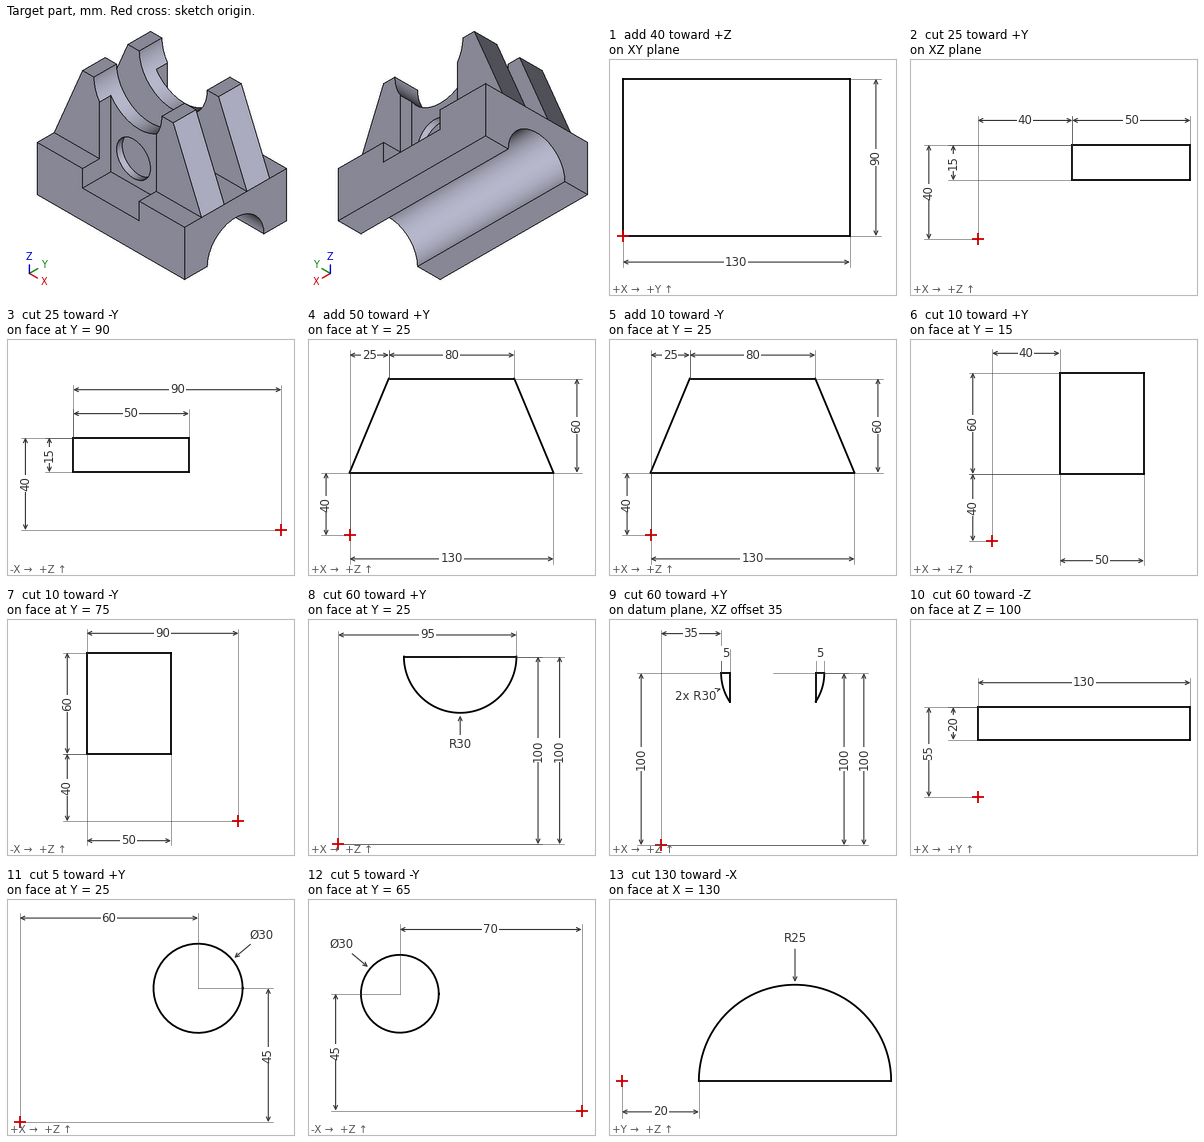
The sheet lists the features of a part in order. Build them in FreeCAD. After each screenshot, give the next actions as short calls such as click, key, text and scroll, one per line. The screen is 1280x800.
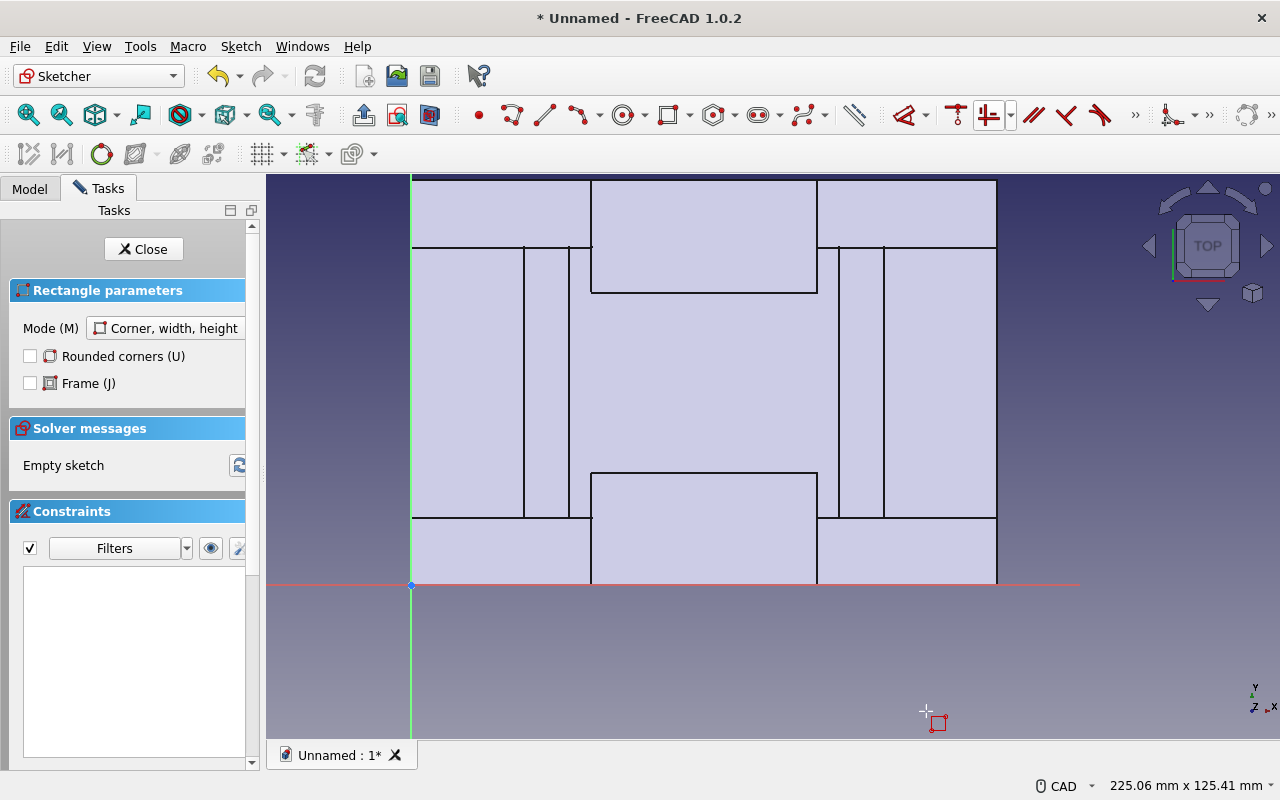
click(411, 338)
click(997, 428)
key(Escape)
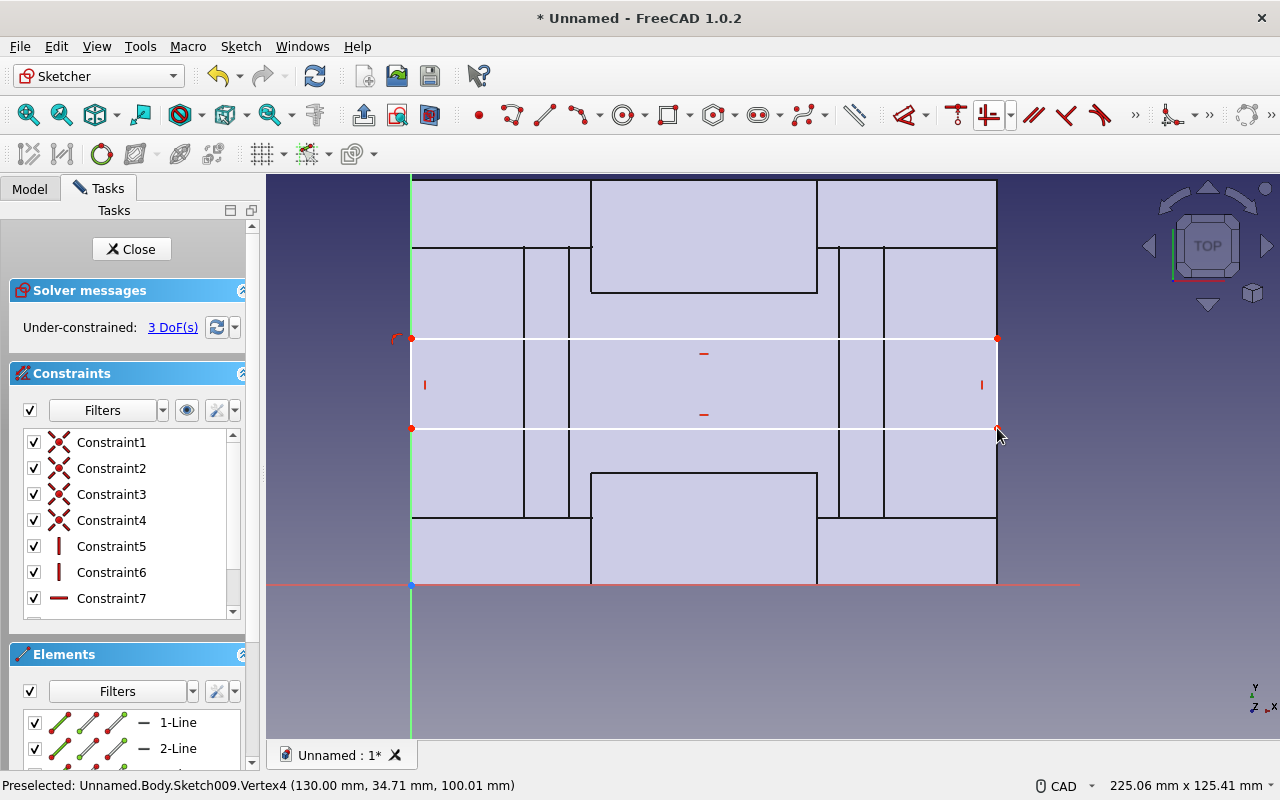
key(d)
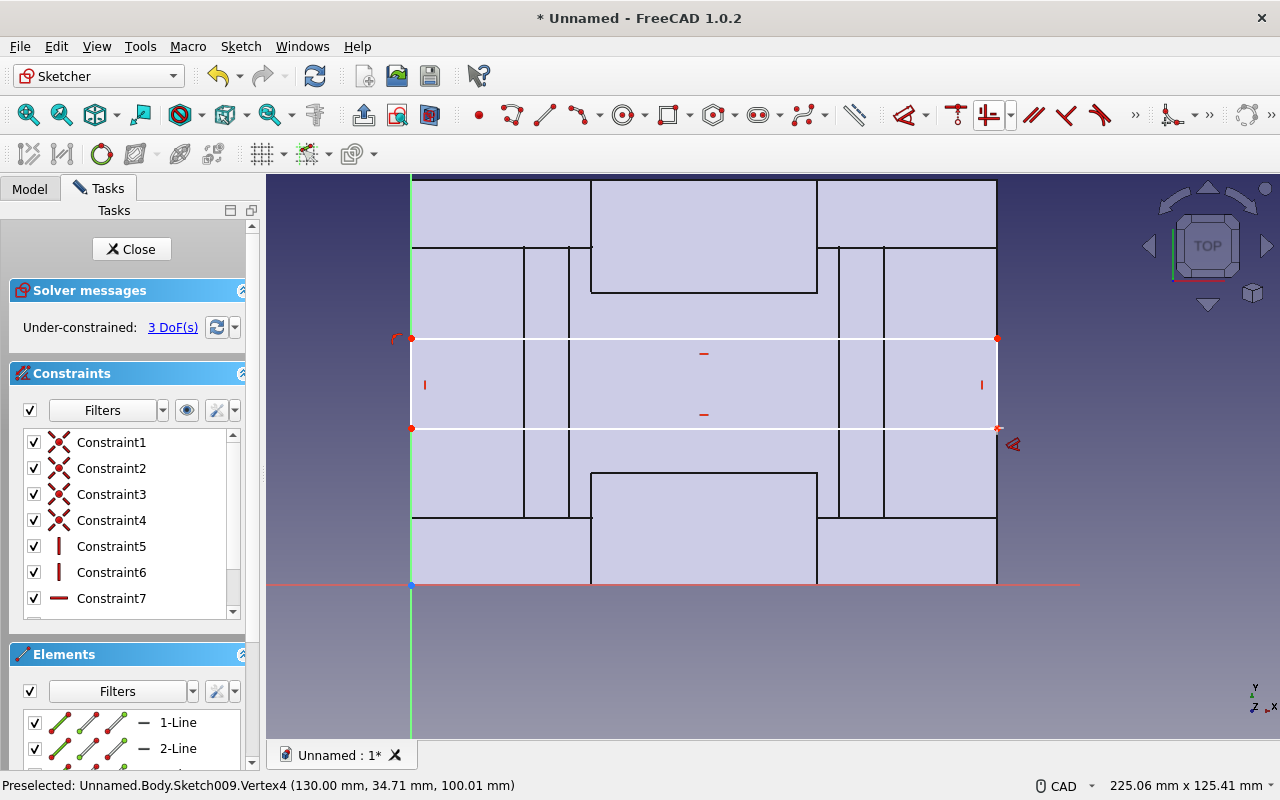
click(411, 366)
click(377, 384)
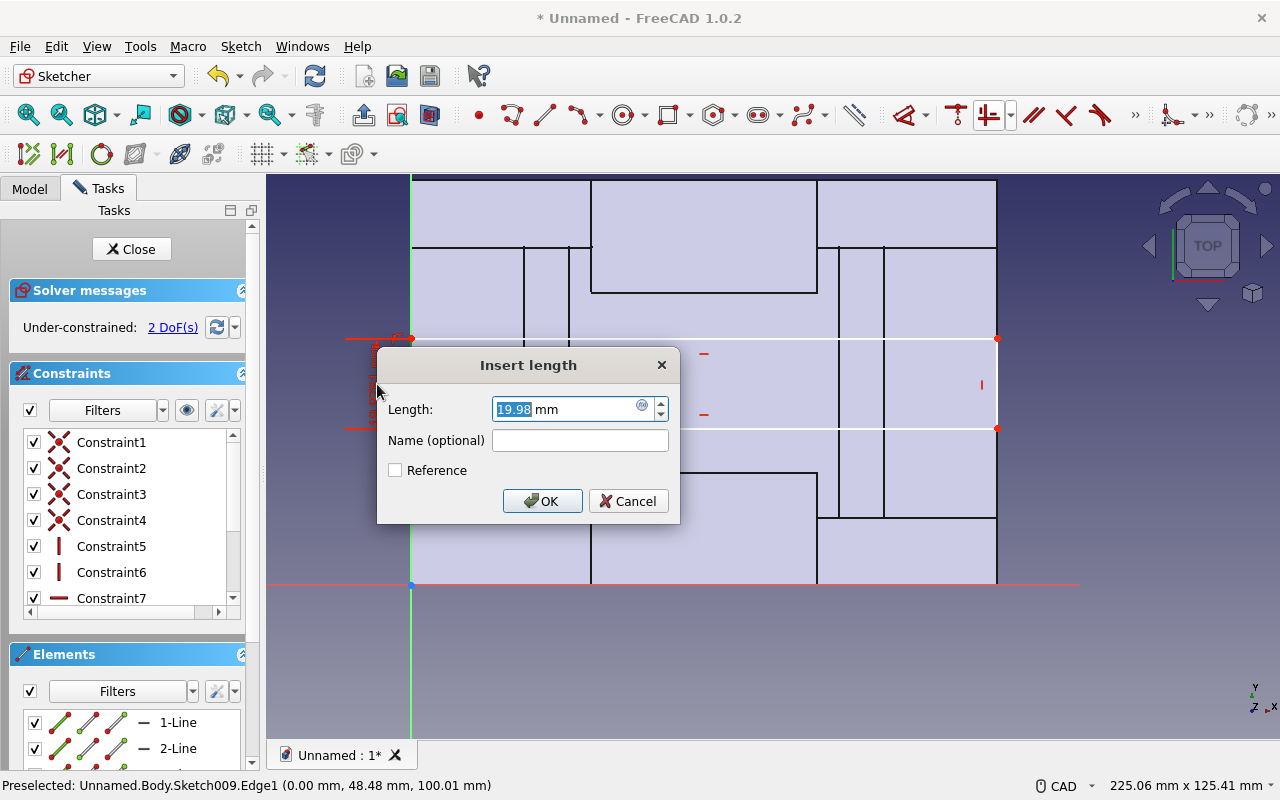
text(20)
key(Return)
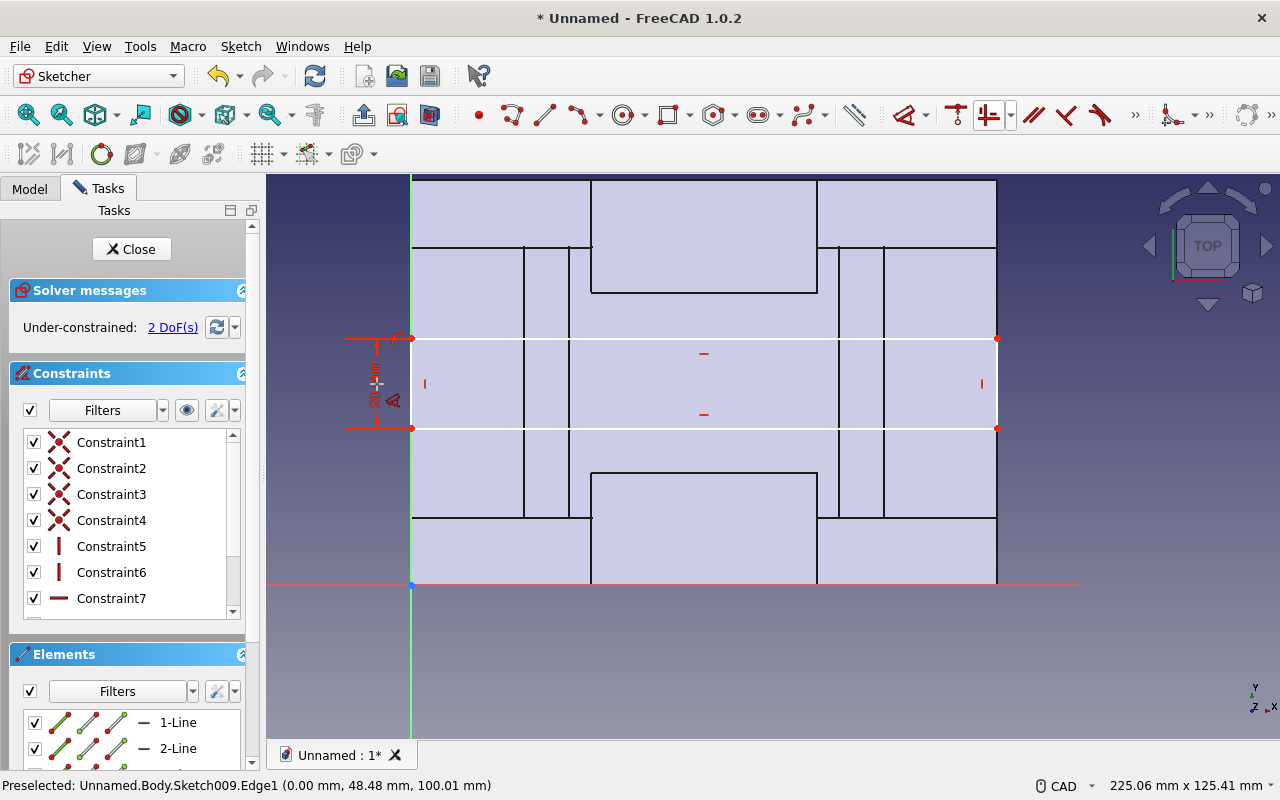
click(587, 429)
click(704, 395)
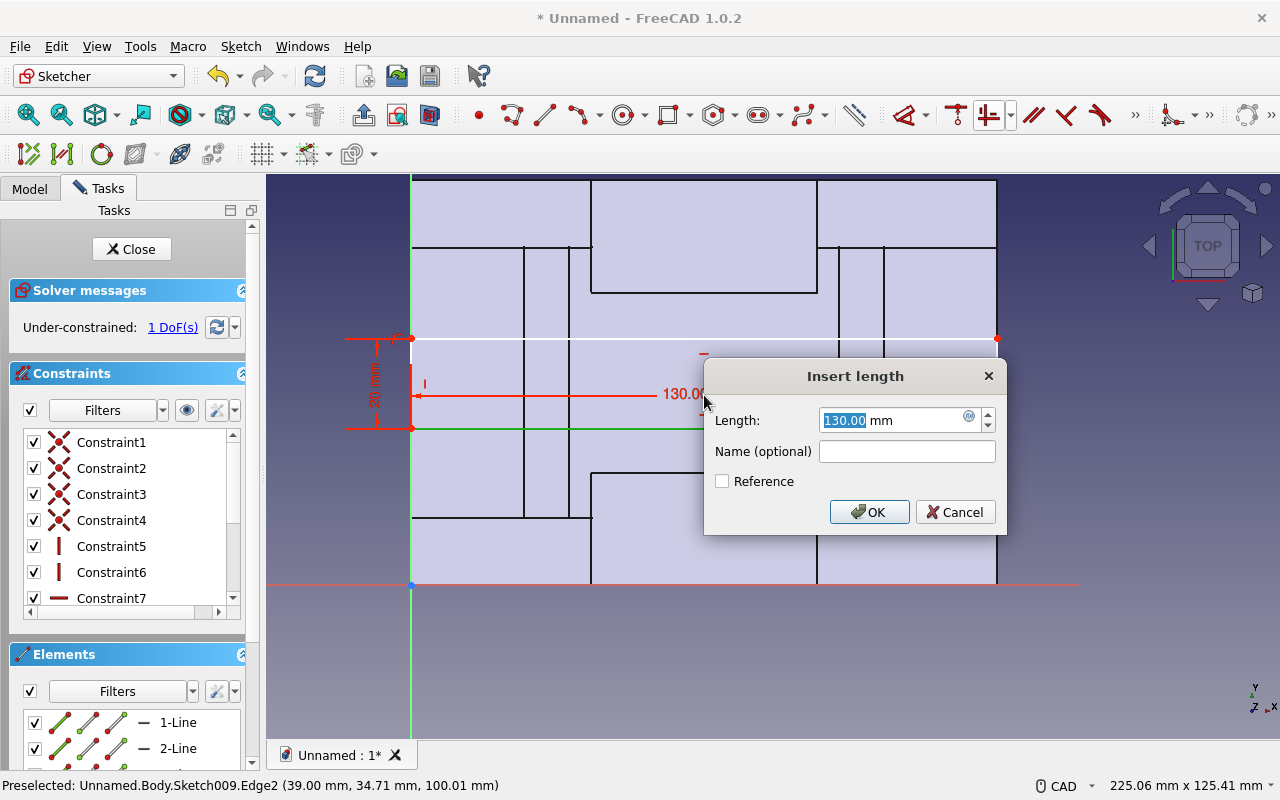
text(130)
key(Return)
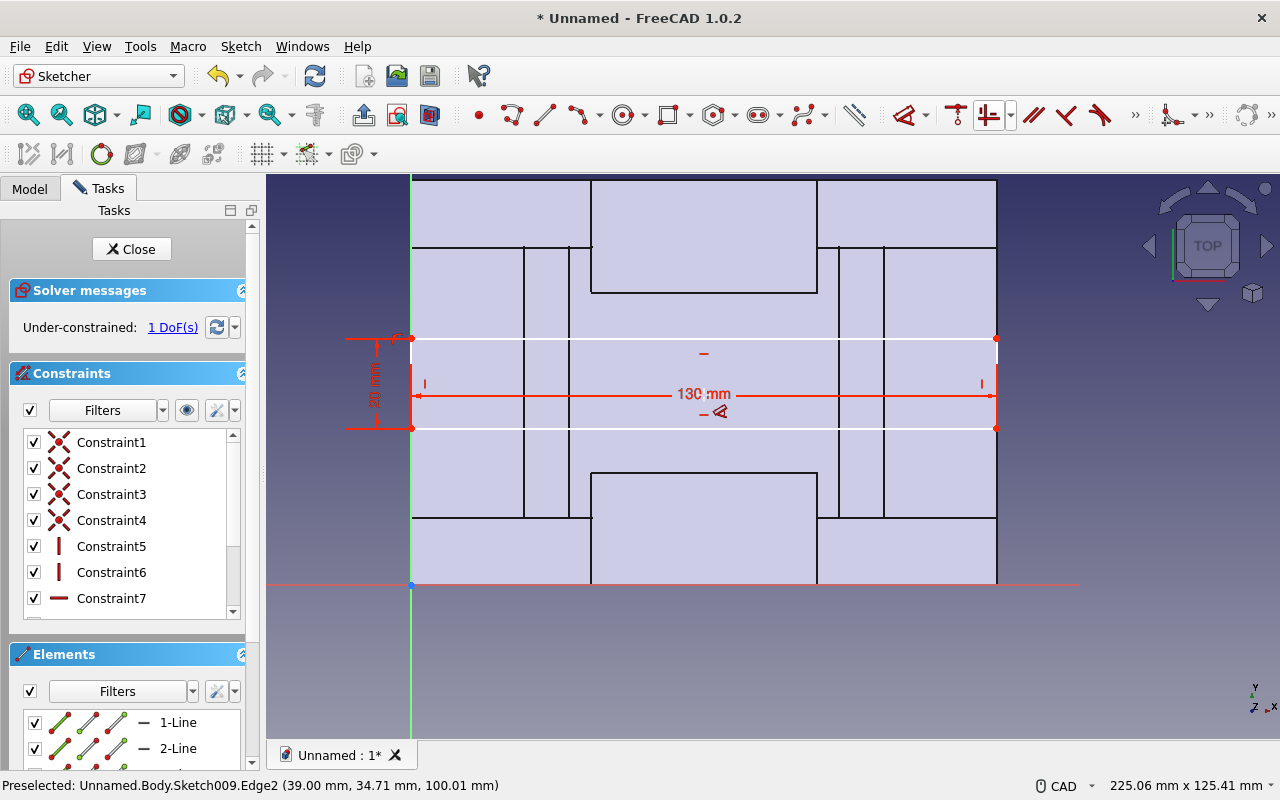
click(411, 339)
click(377, 462)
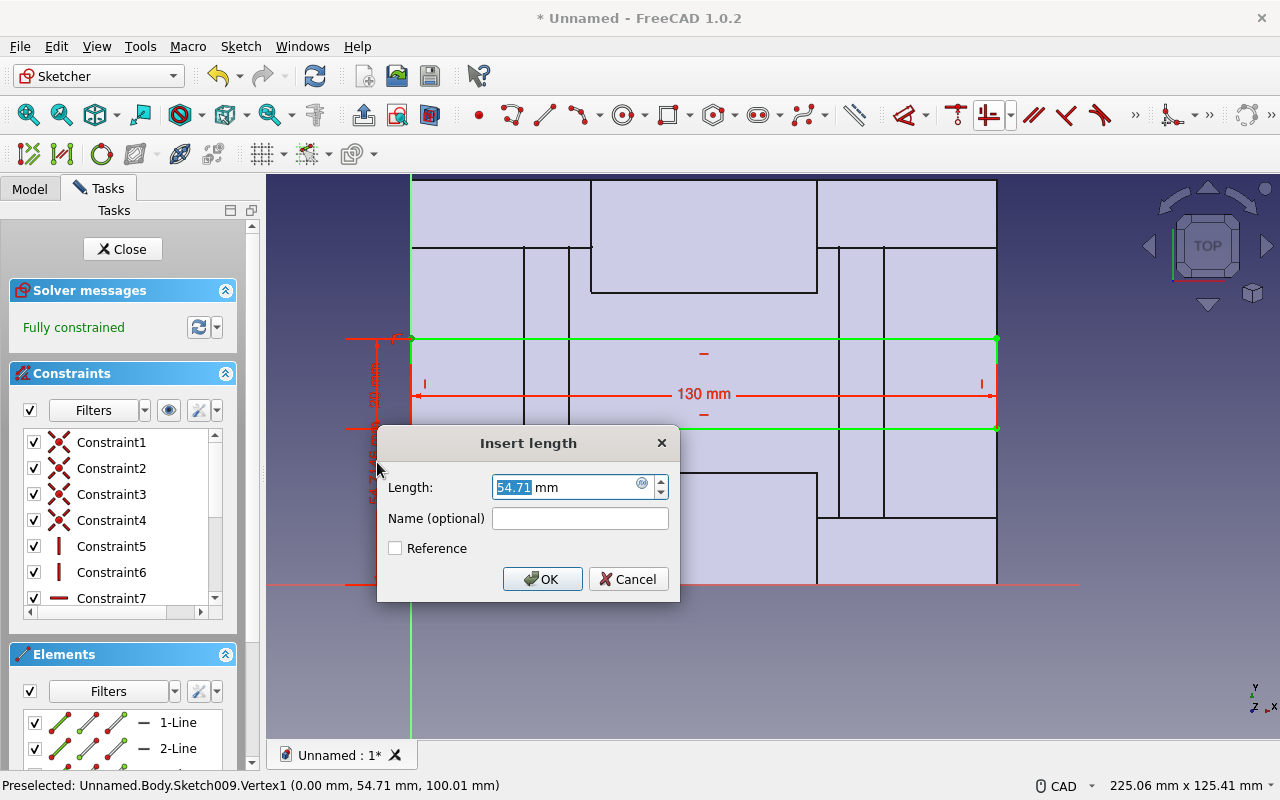
text(55)
key(Return)
key(Escape)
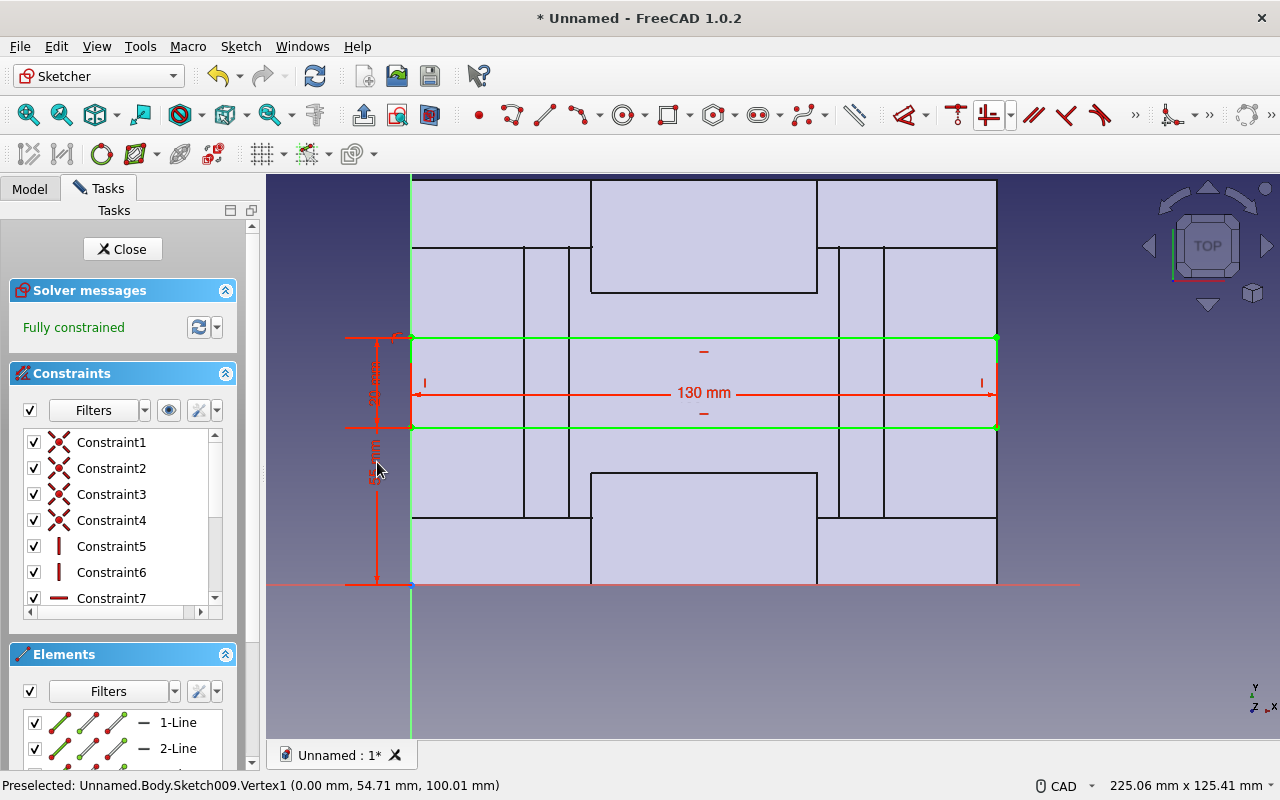
click(123, 249)